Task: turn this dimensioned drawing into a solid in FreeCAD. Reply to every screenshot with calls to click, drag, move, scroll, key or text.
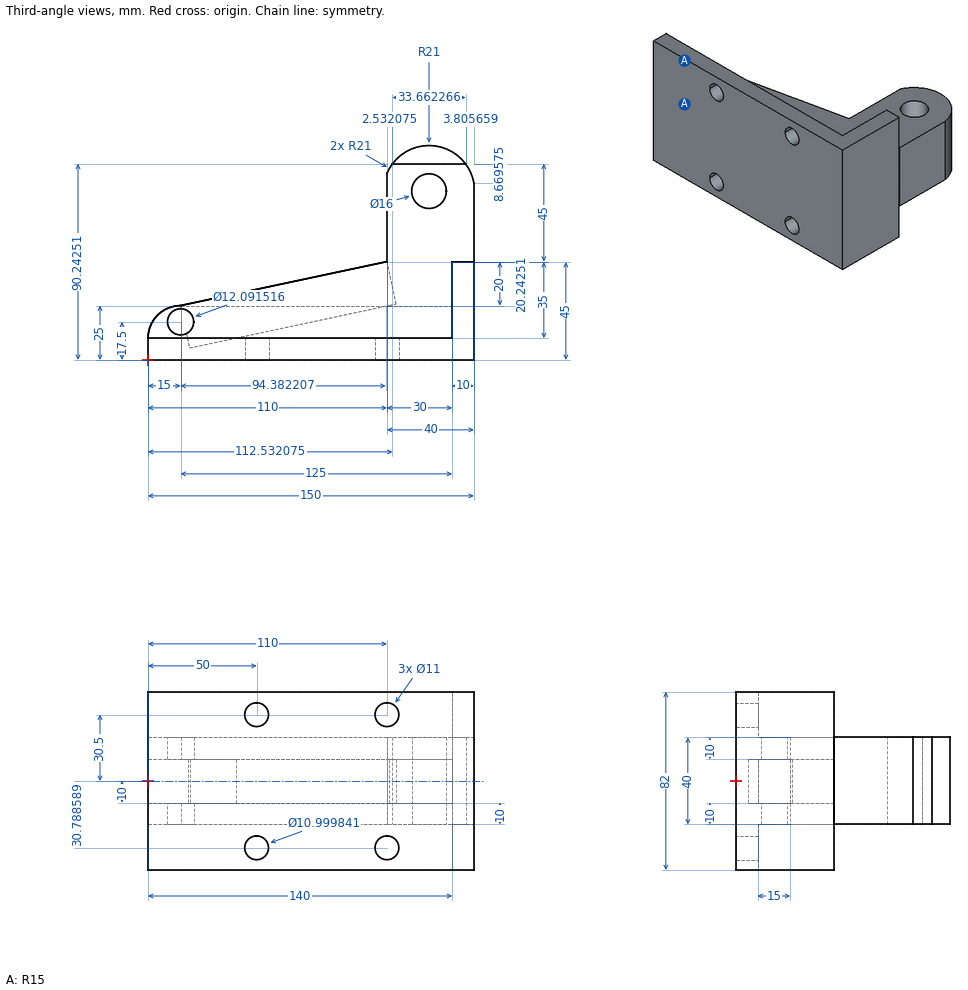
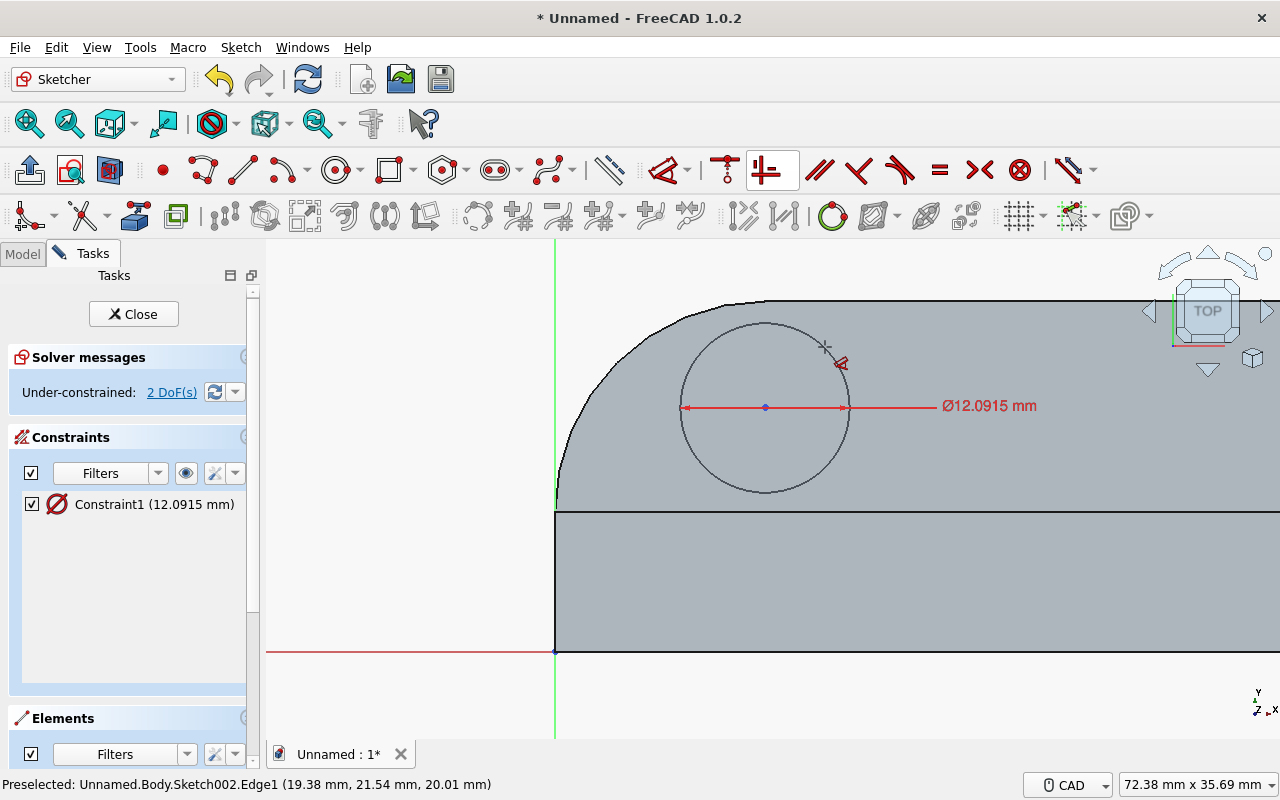
click(765, 408)
click(660, 686)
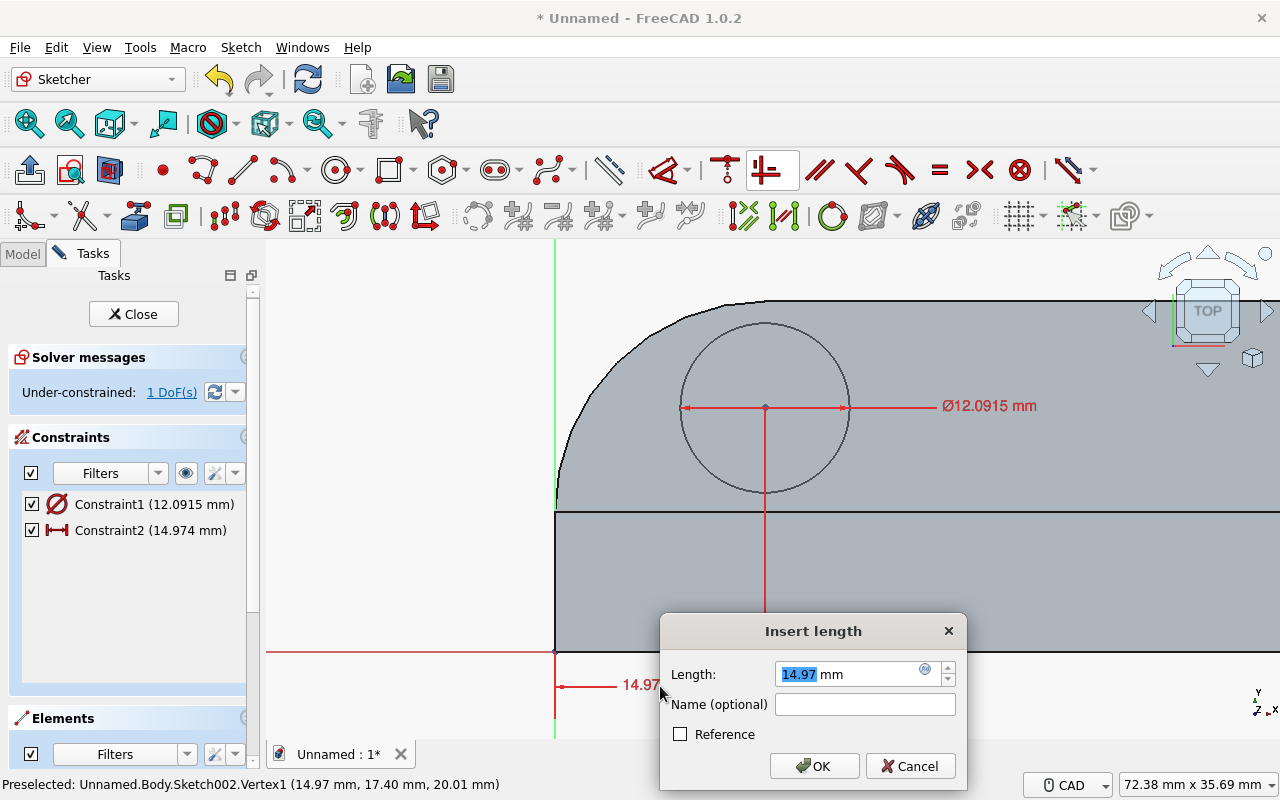
text(15)
key(Return)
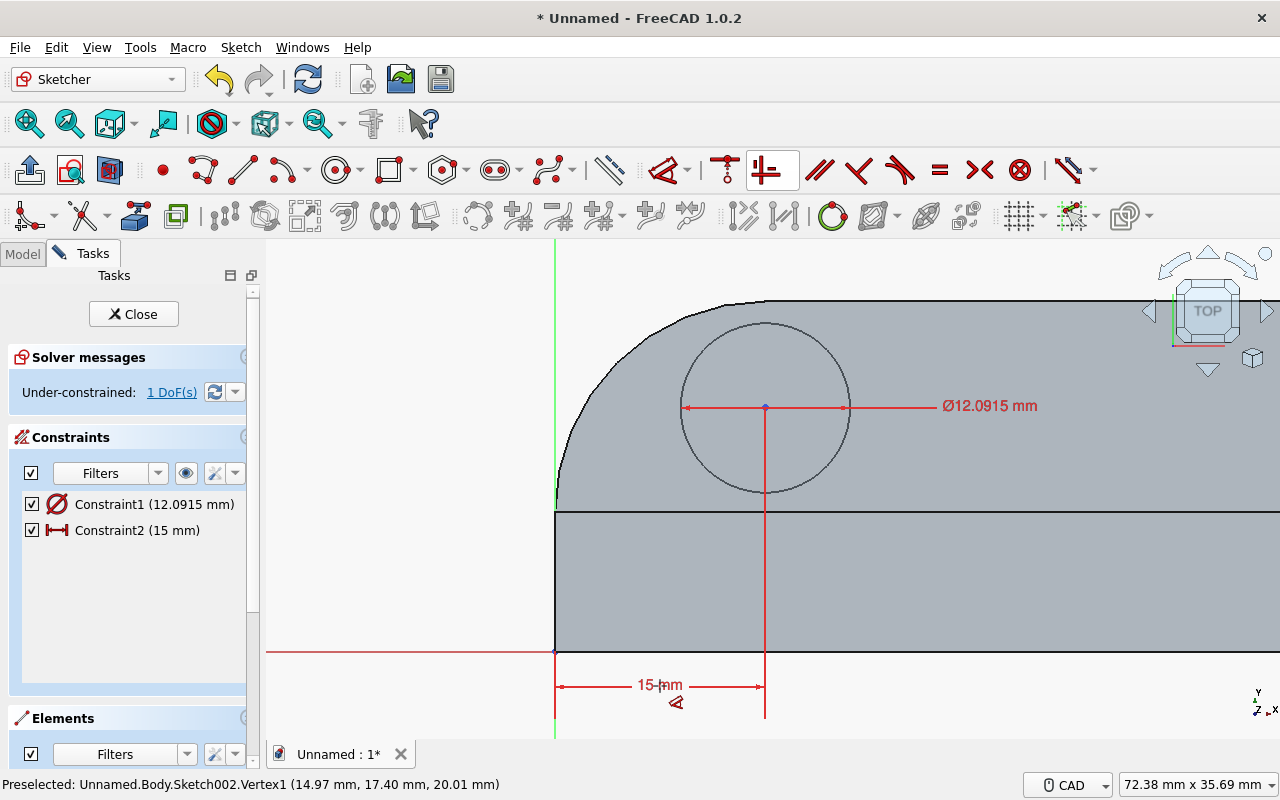
click(765, 408)
click(521, 530)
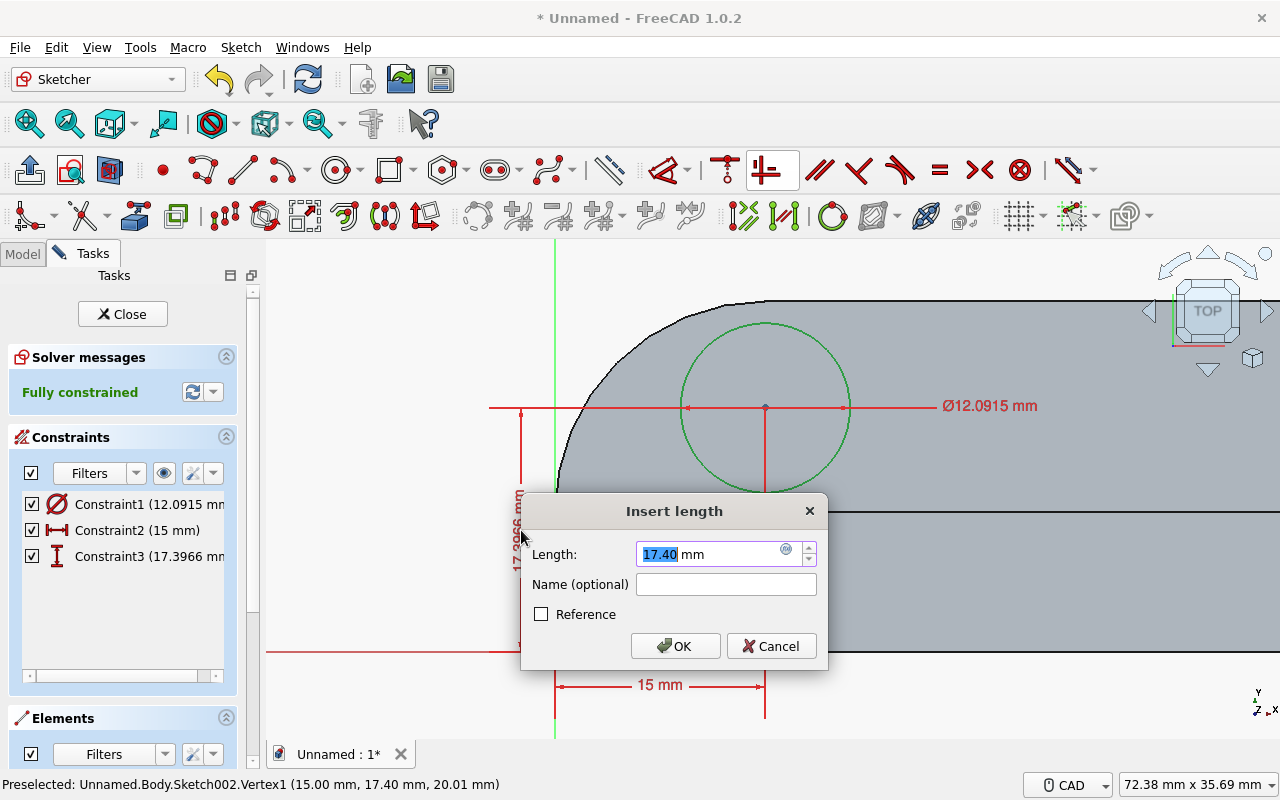
text(17.5)
key(Return)
key(Escape)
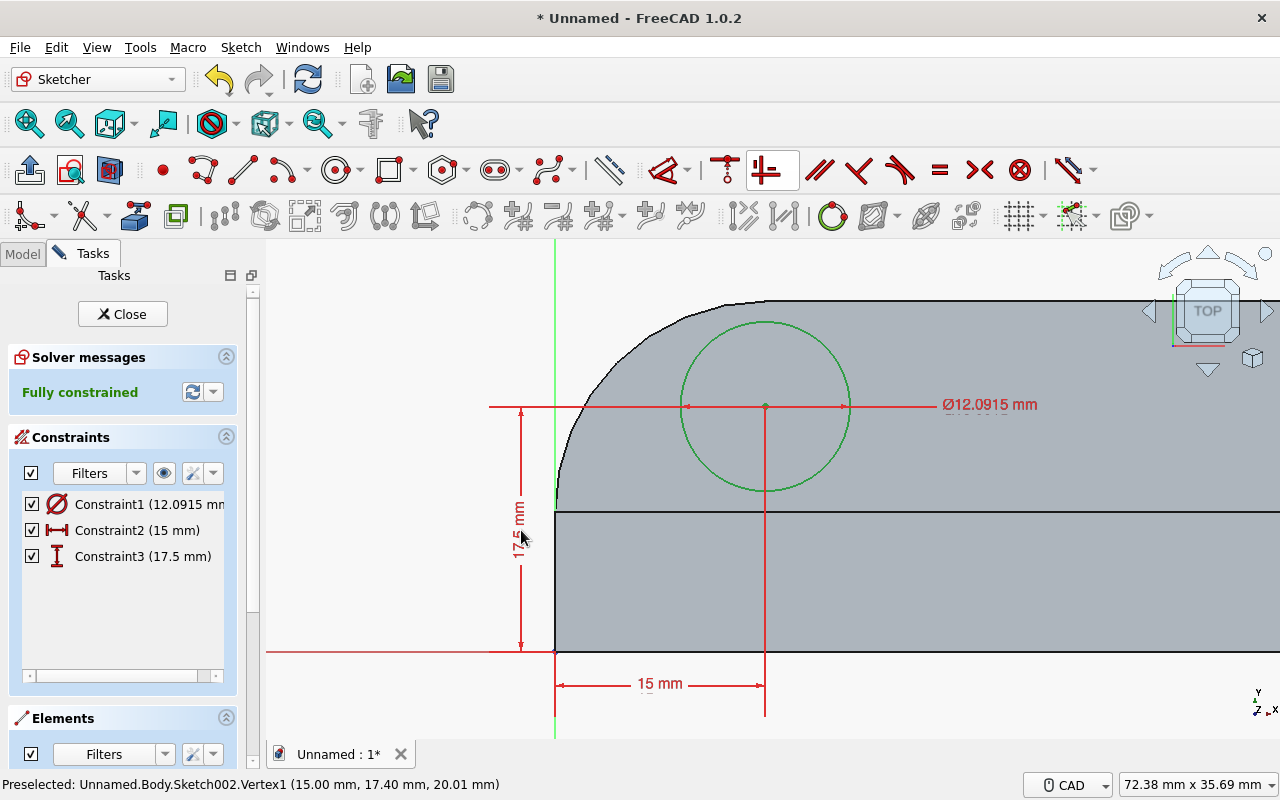
click(123, 314)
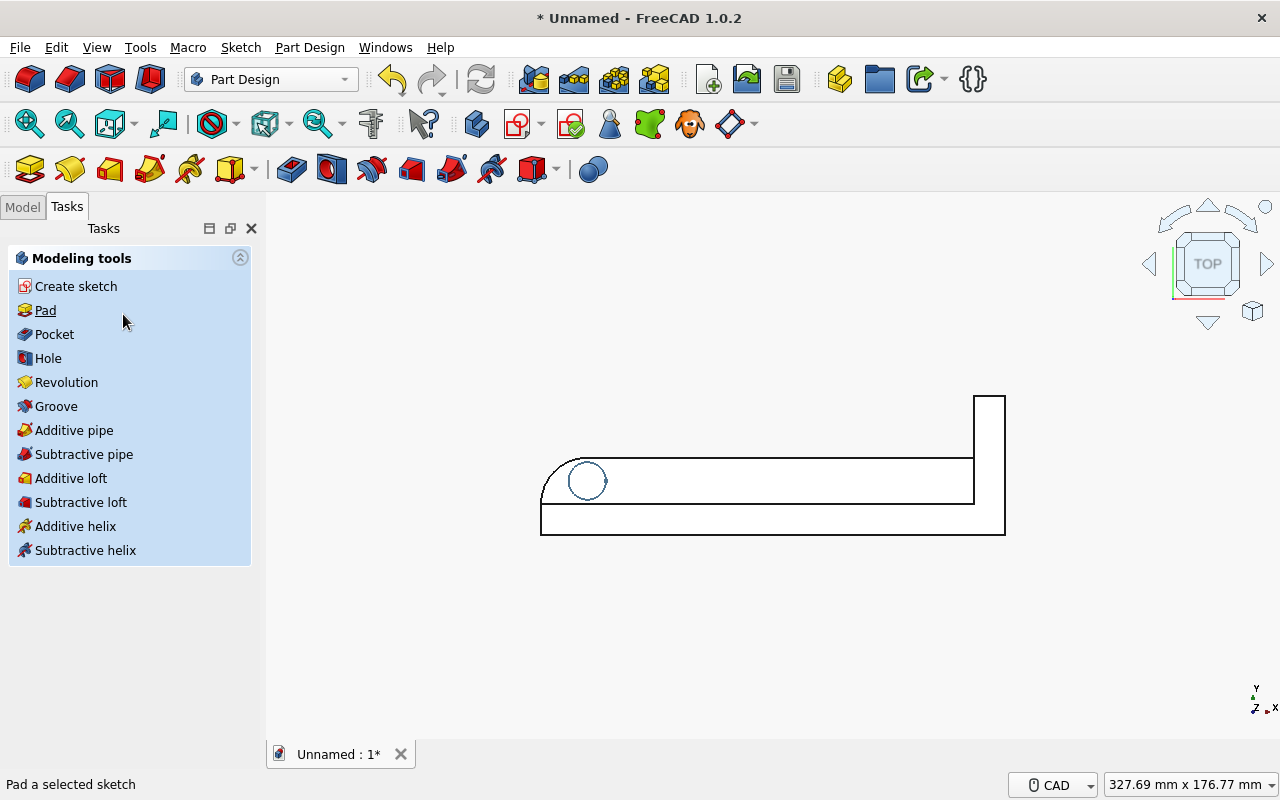
click(292, 170)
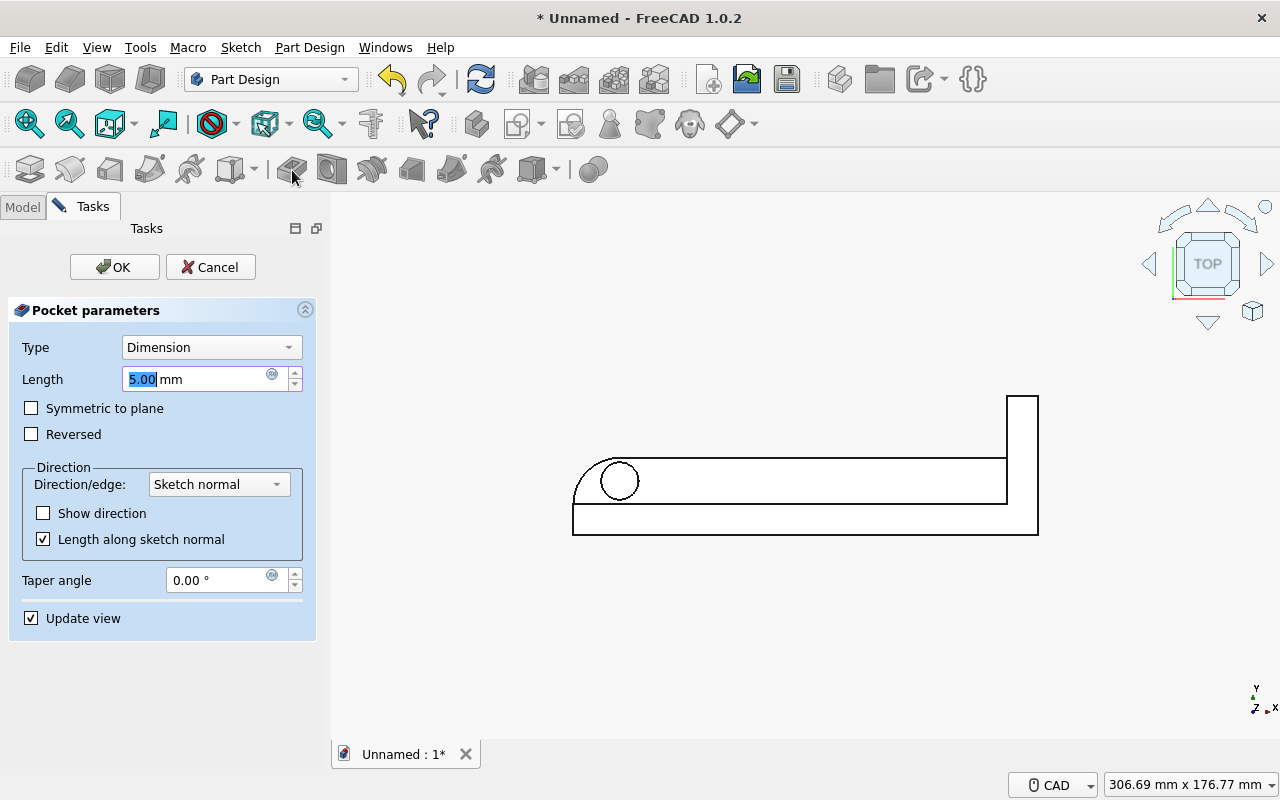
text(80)
key(Tab)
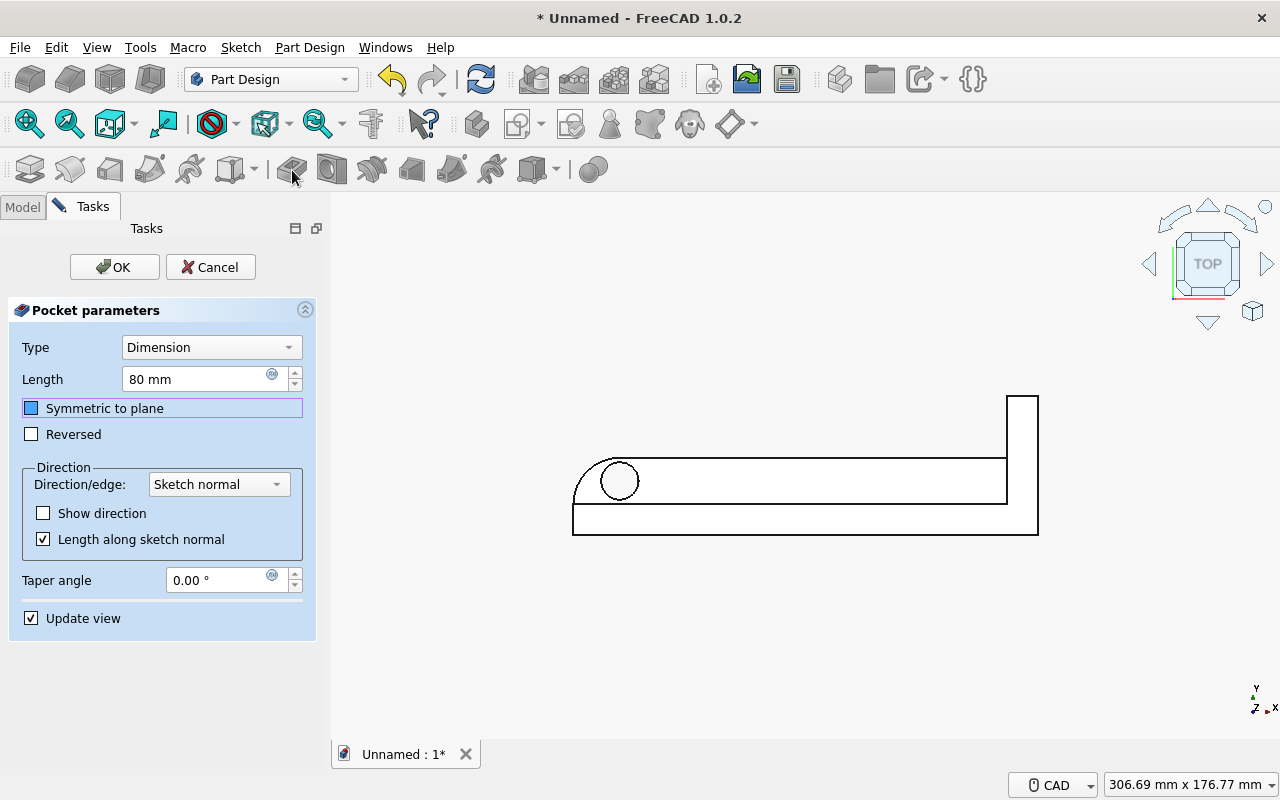
click(115, 267)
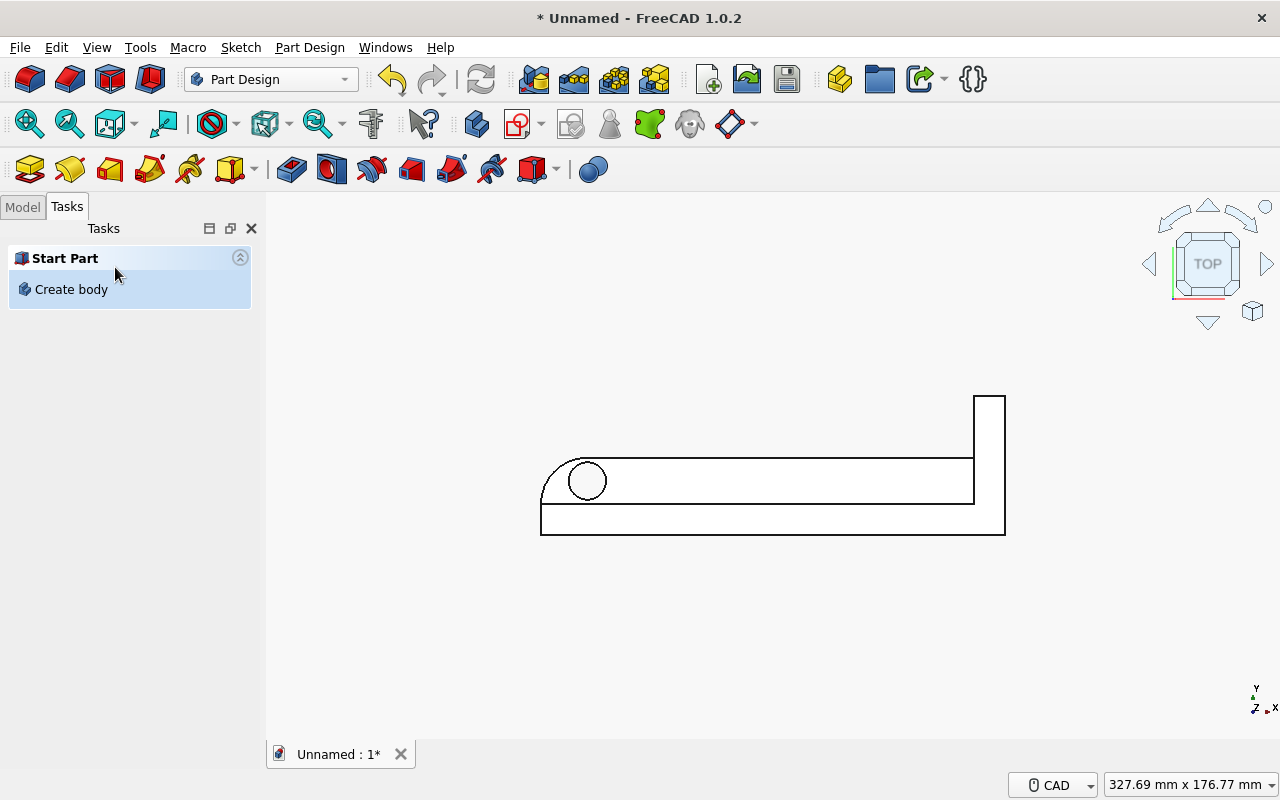
key(4)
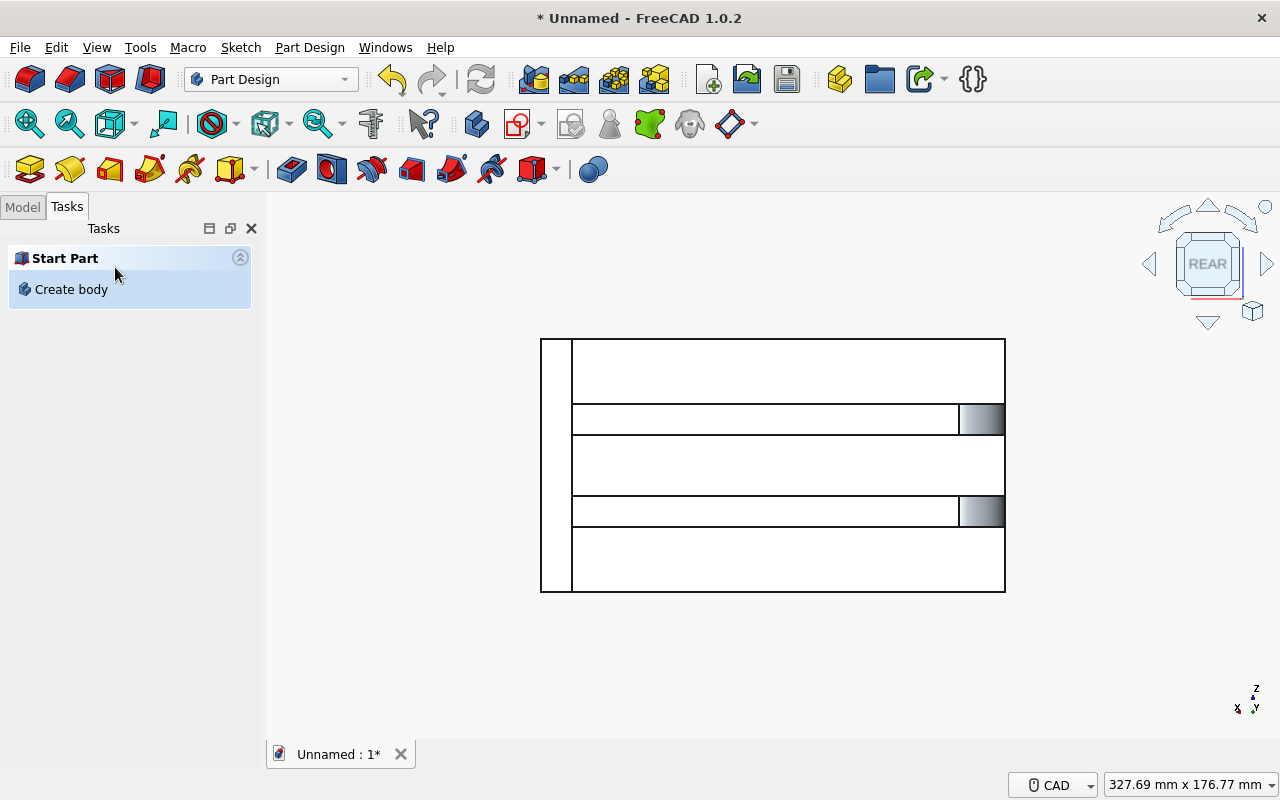
click(665, 559)